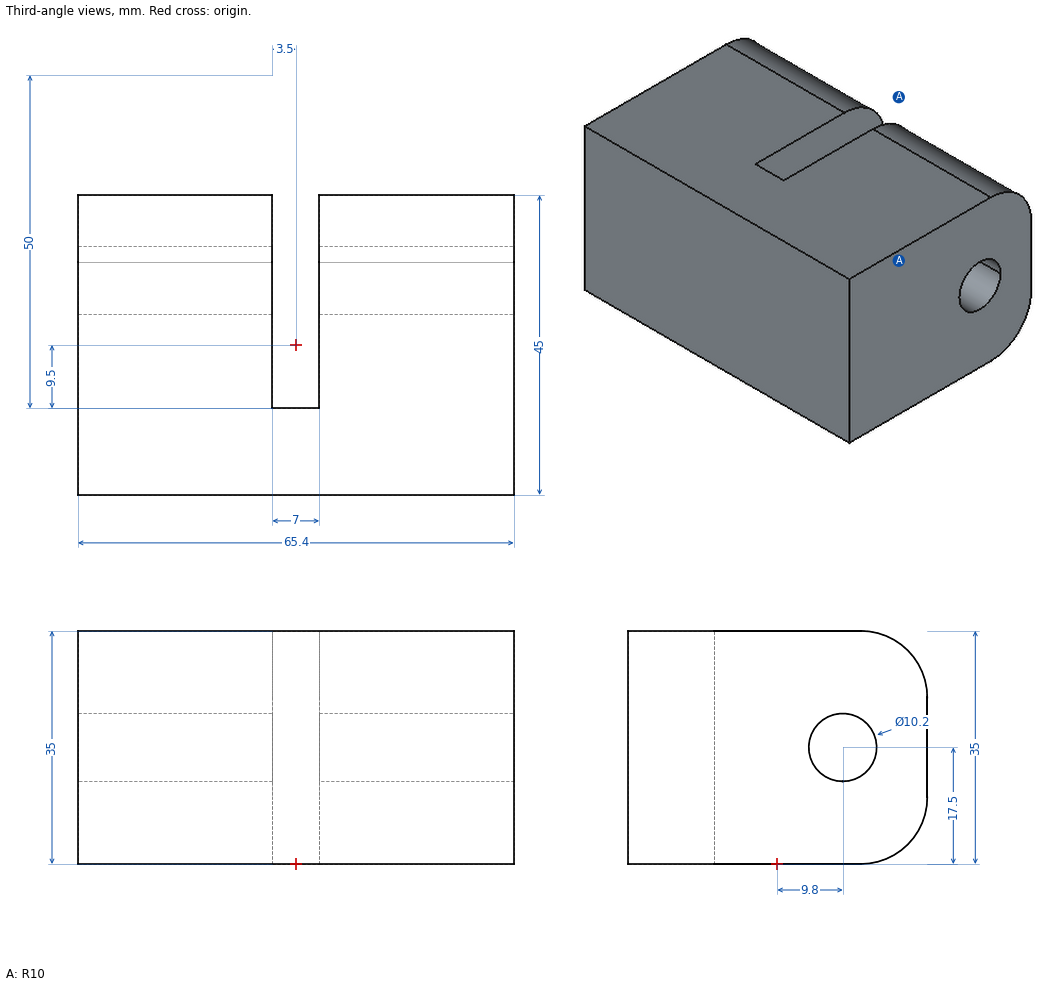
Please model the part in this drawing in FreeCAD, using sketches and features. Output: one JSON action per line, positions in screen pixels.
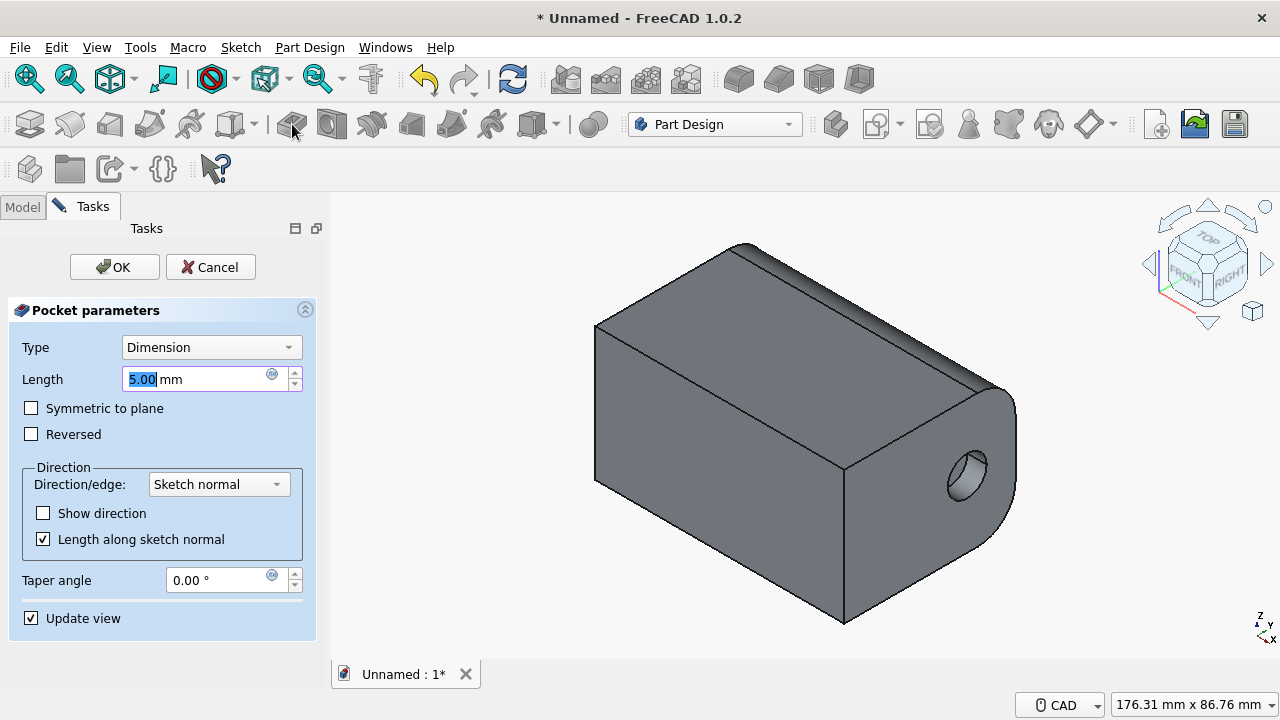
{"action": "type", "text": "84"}
{"action": "key", "text": "Tab"}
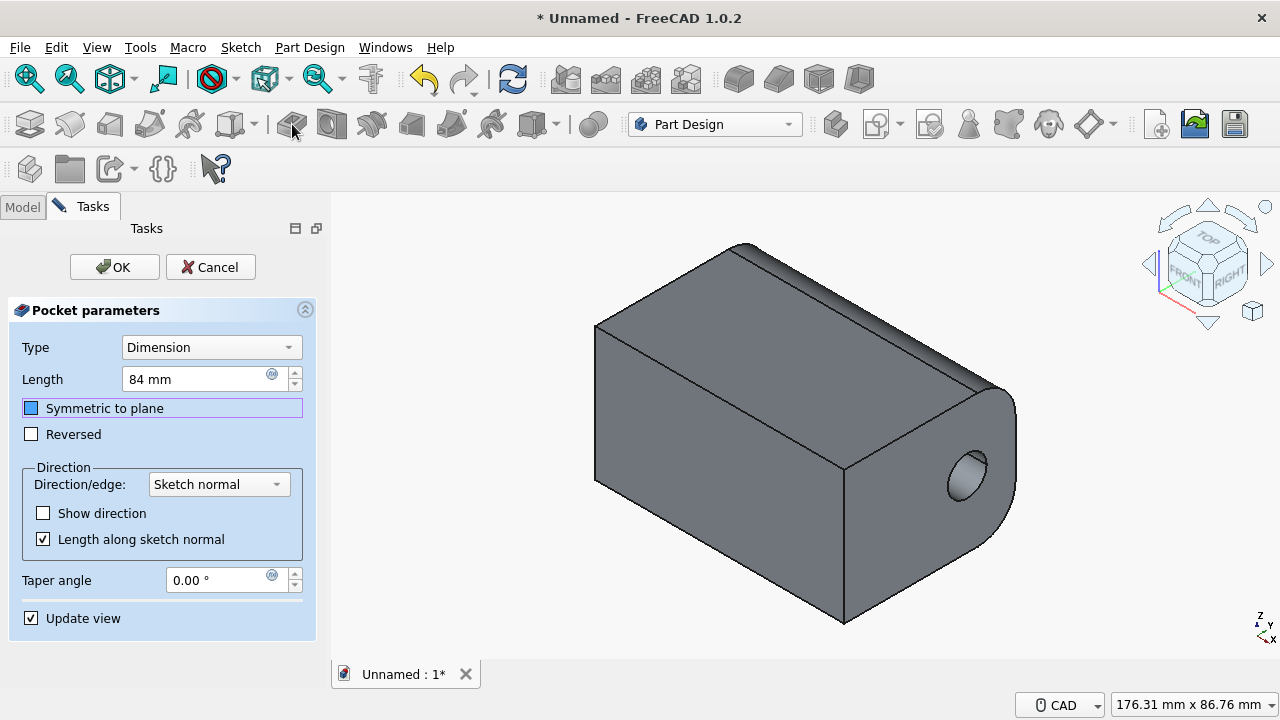
{"action": "left_click", "coordinate": [115, 267]}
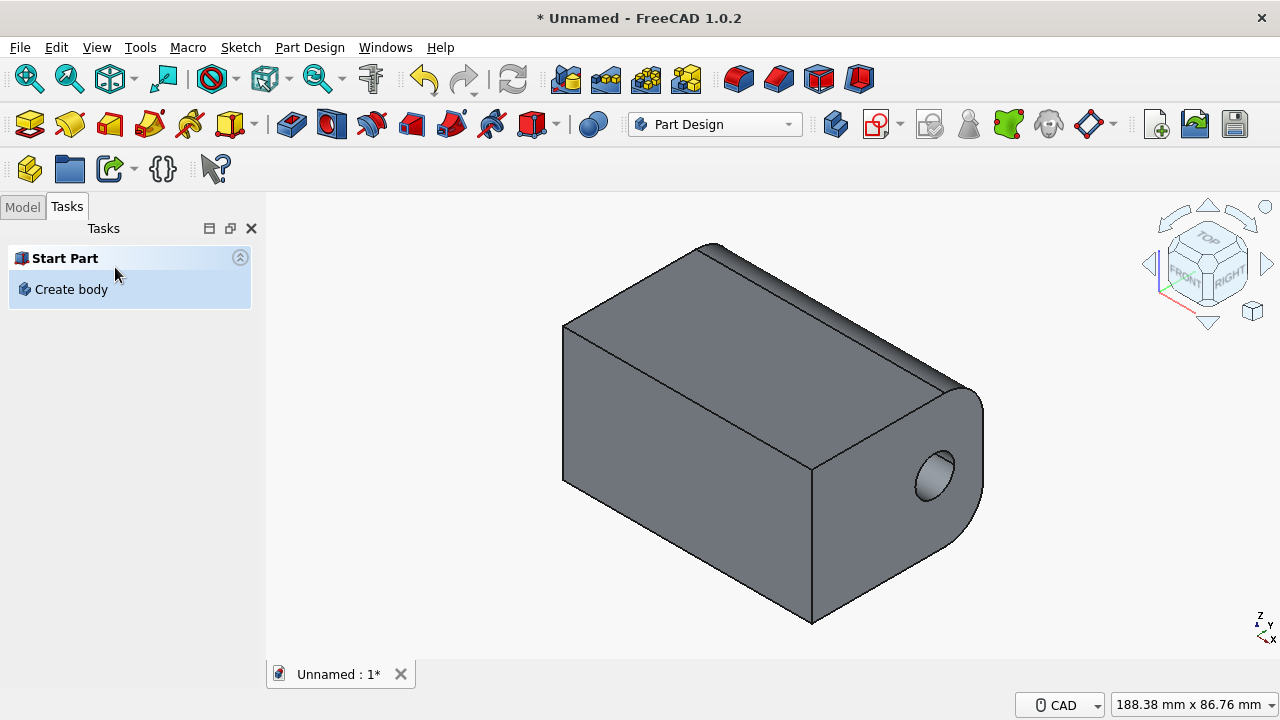
{"action": "left_click", "coordinate": [790, 379]}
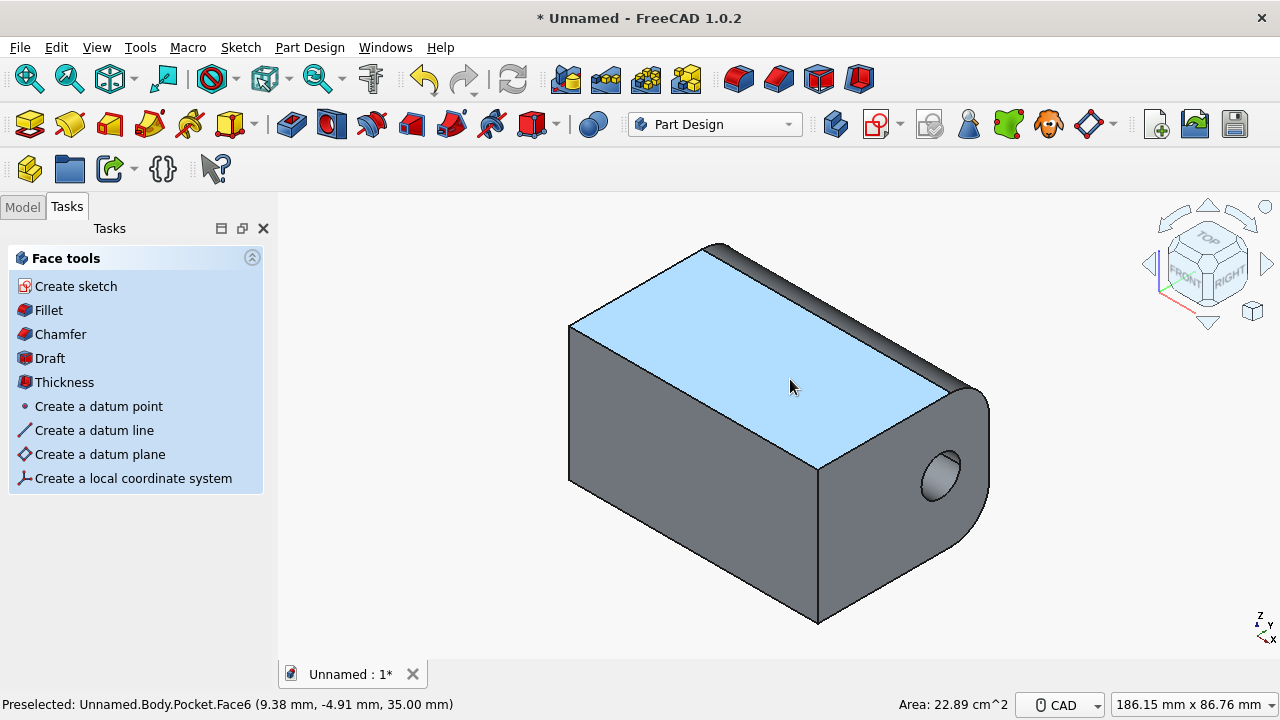
{"action": "left_click", "coordinate": [876, 124]}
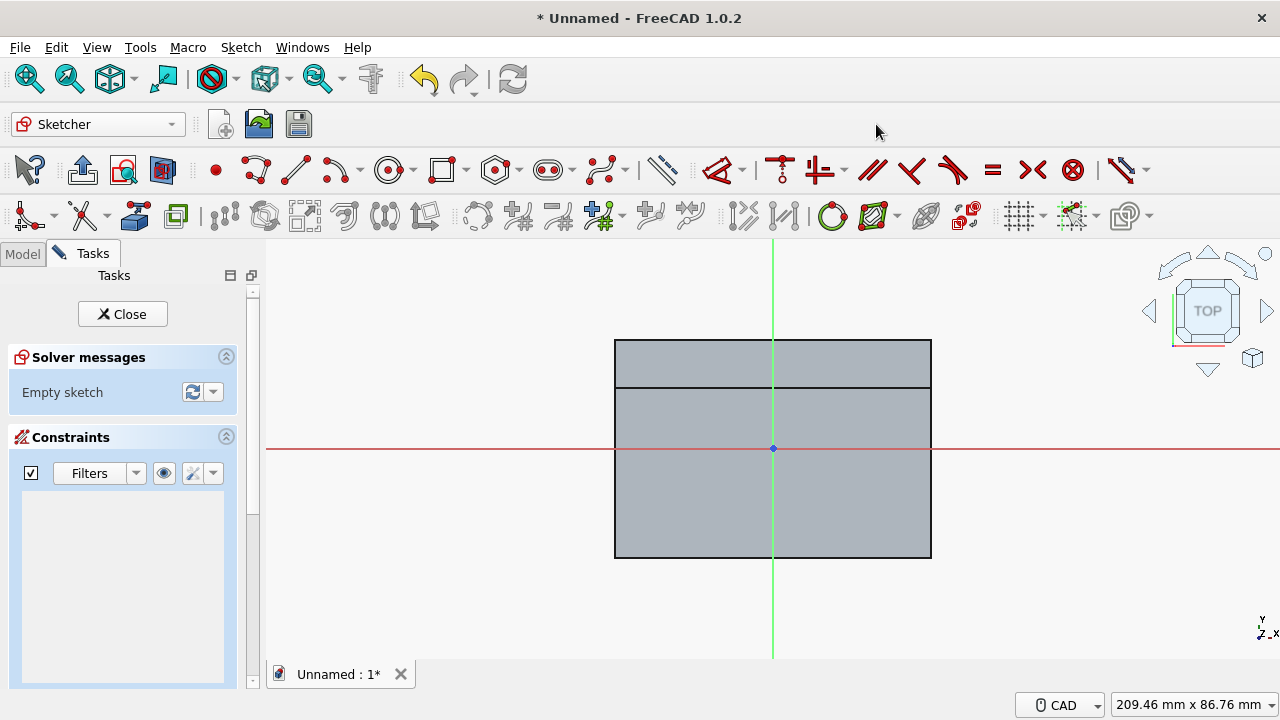
{"action": "scroll", "coordinate": [395, 631], "scroll_direction": "down", "scroll_amount": 1}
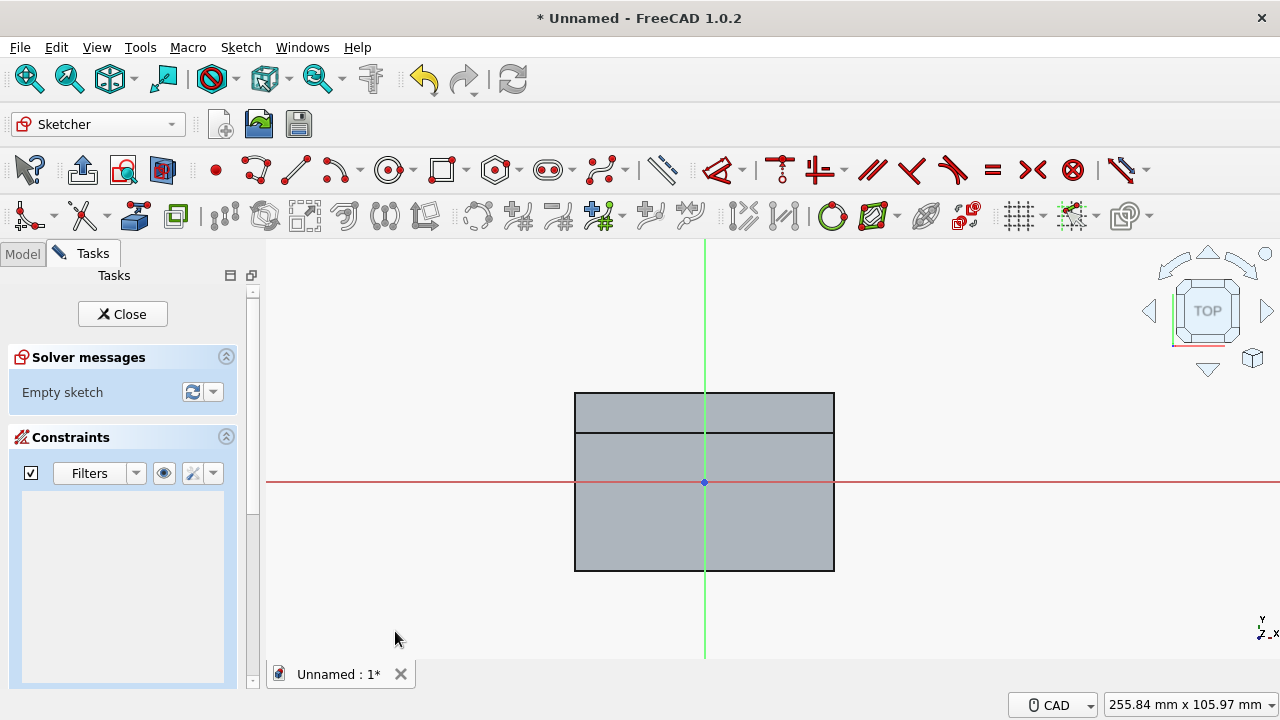
{"action": "left_click", "coordinate": [442, 170]}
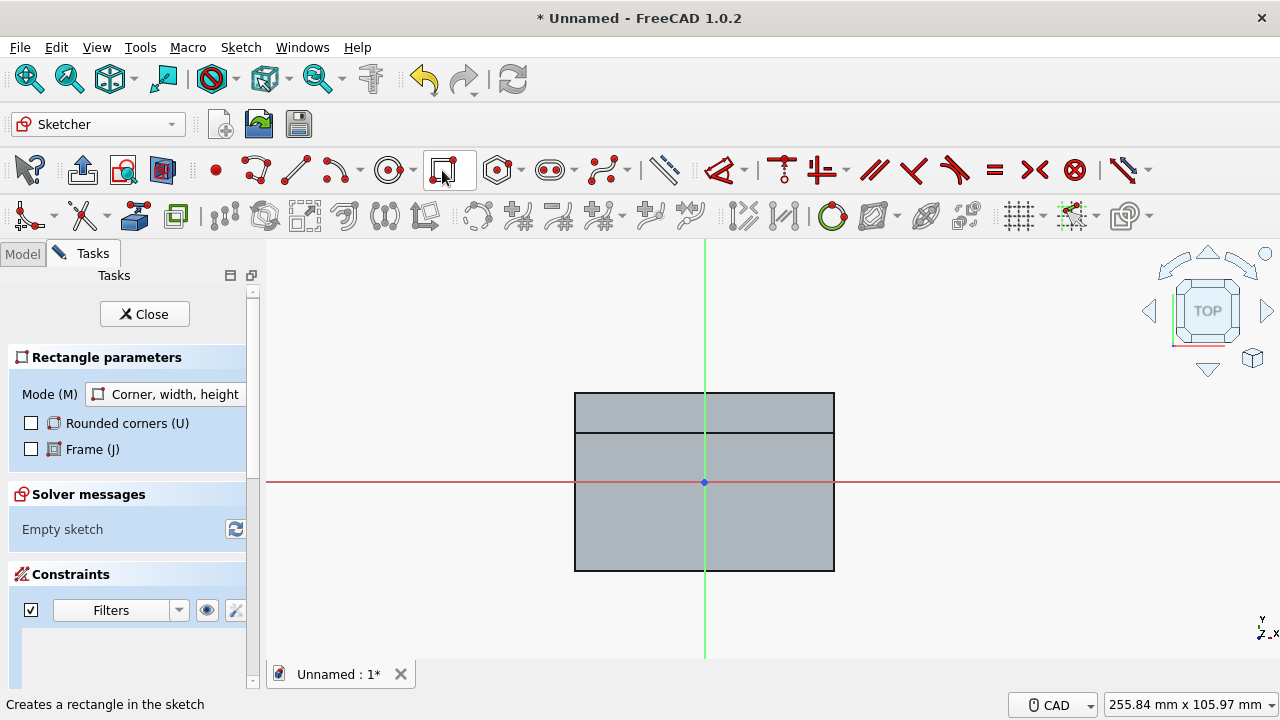
{"action": "left_click", "coordinate": [691, 322]}
{"action": "left_click", "coordinate": [718, 520]}
{"action": "key", "text": "Escape"}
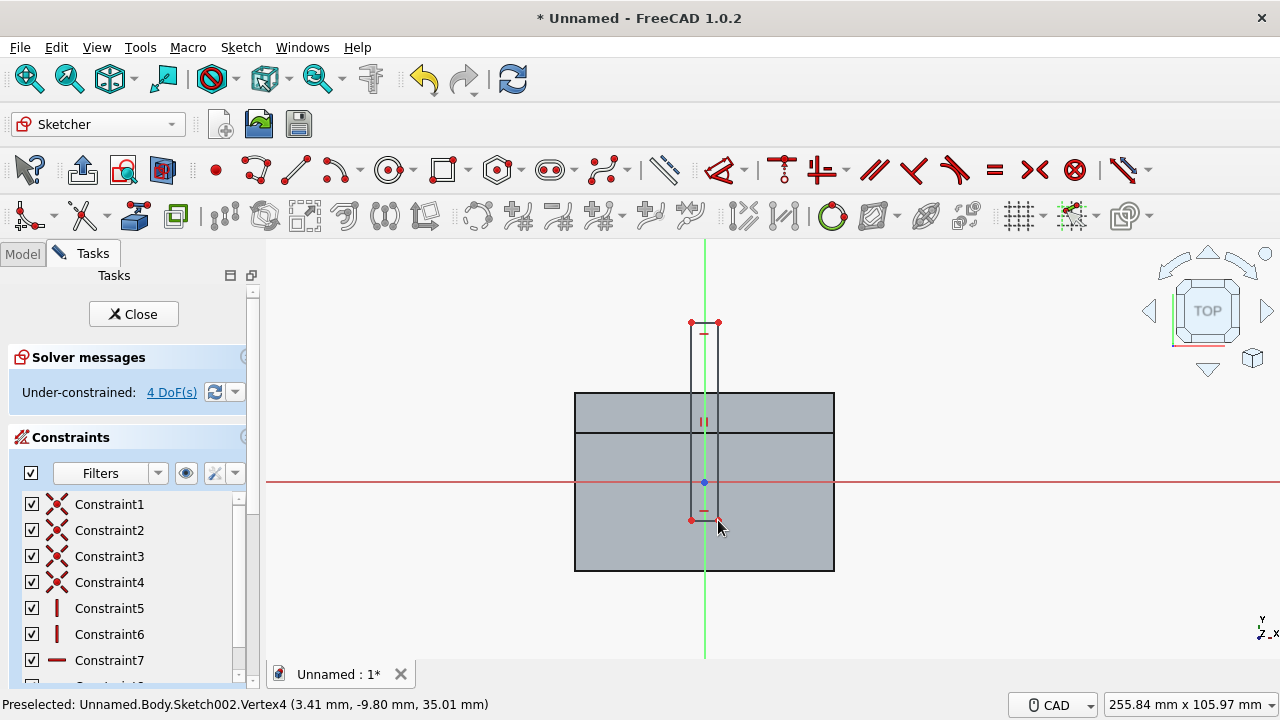
{"action": "left_click", "coordinate": [720, 170]}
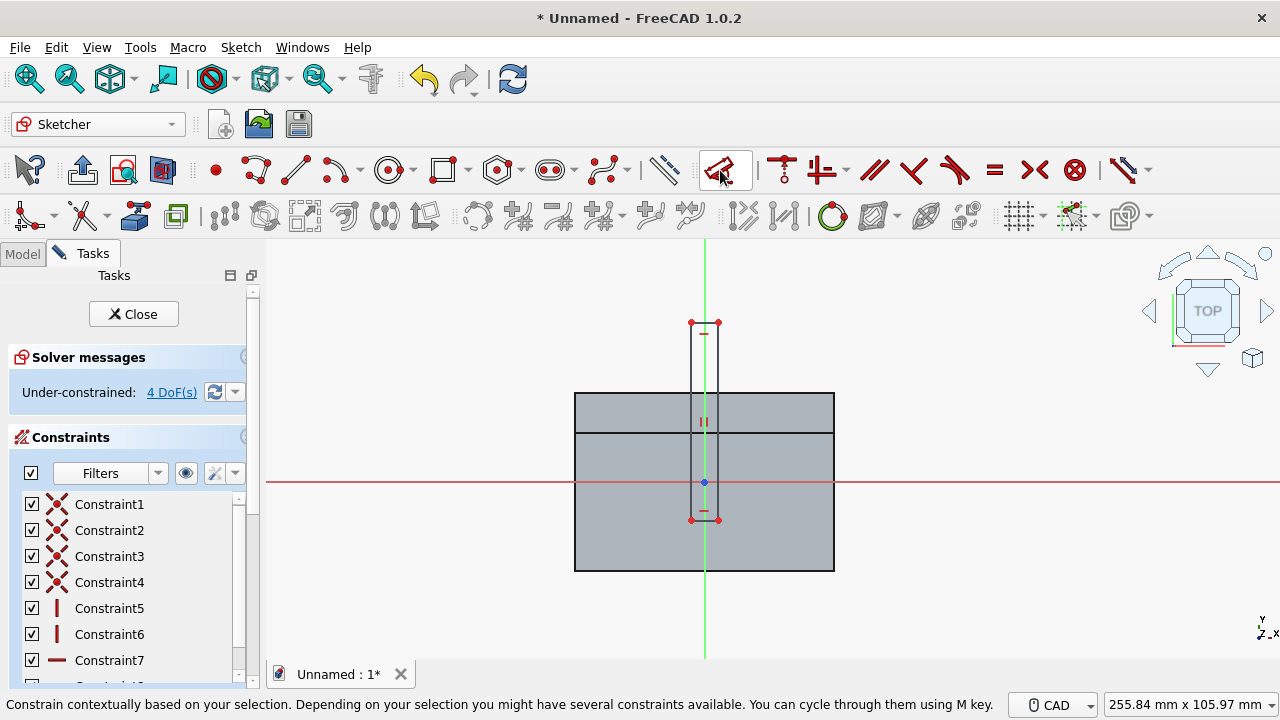
{"action": "scroll", "coordinate": [702, 521], "scroll_direction": "up", "scroll_amount": 2}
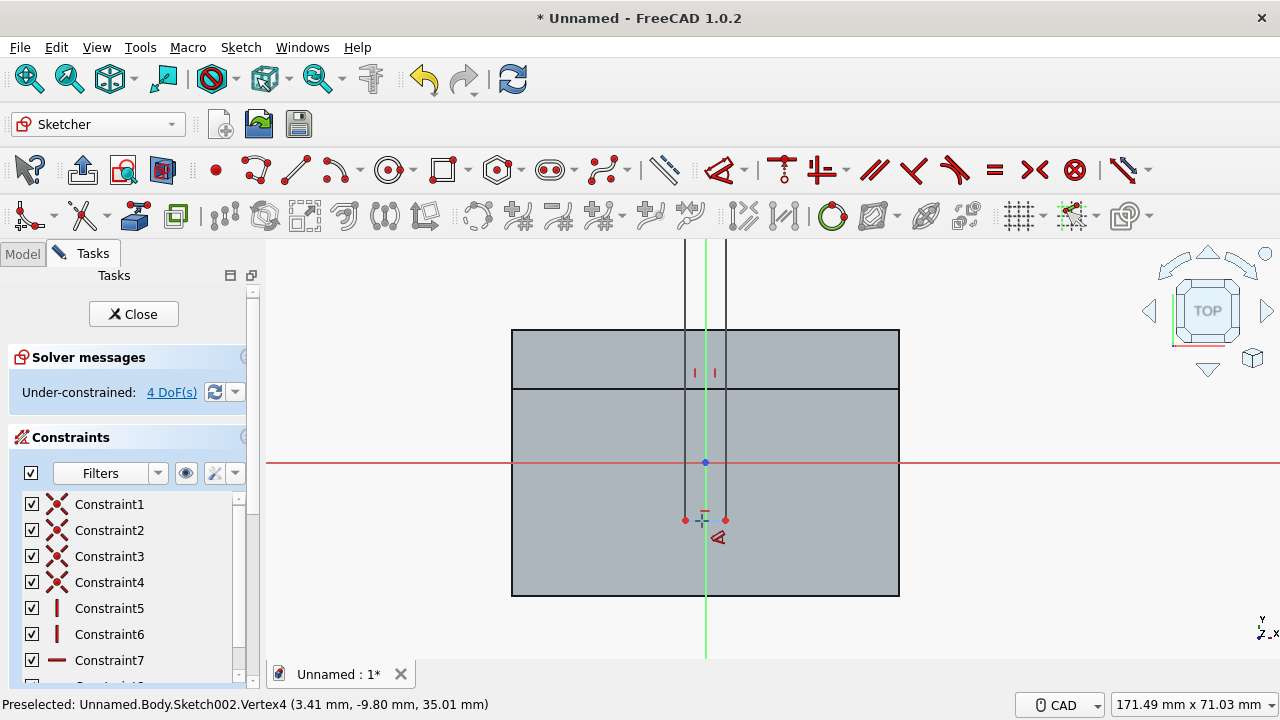
{"action": "left_click", "coordinate": [701, 521]}
{"action": "left_click", "coordinate": [691, 555]}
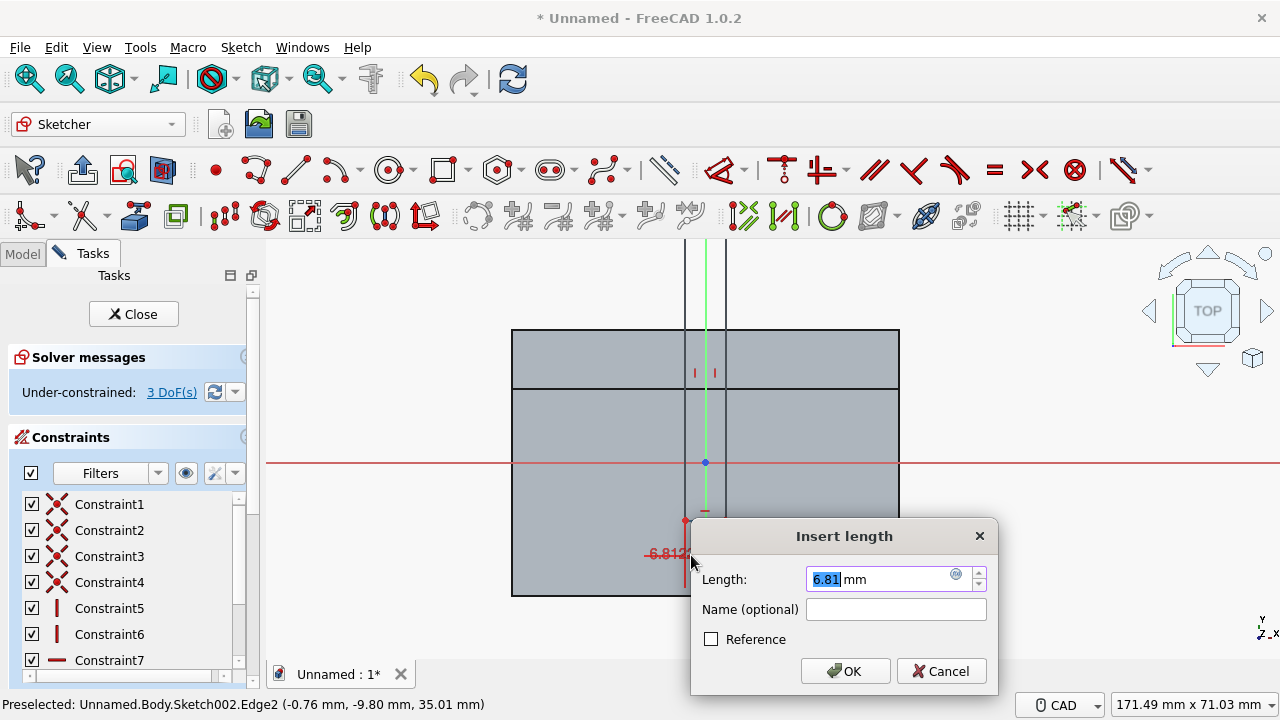
{"action": "type", "text": "7"}
{"action": "key", "text": "Return"}